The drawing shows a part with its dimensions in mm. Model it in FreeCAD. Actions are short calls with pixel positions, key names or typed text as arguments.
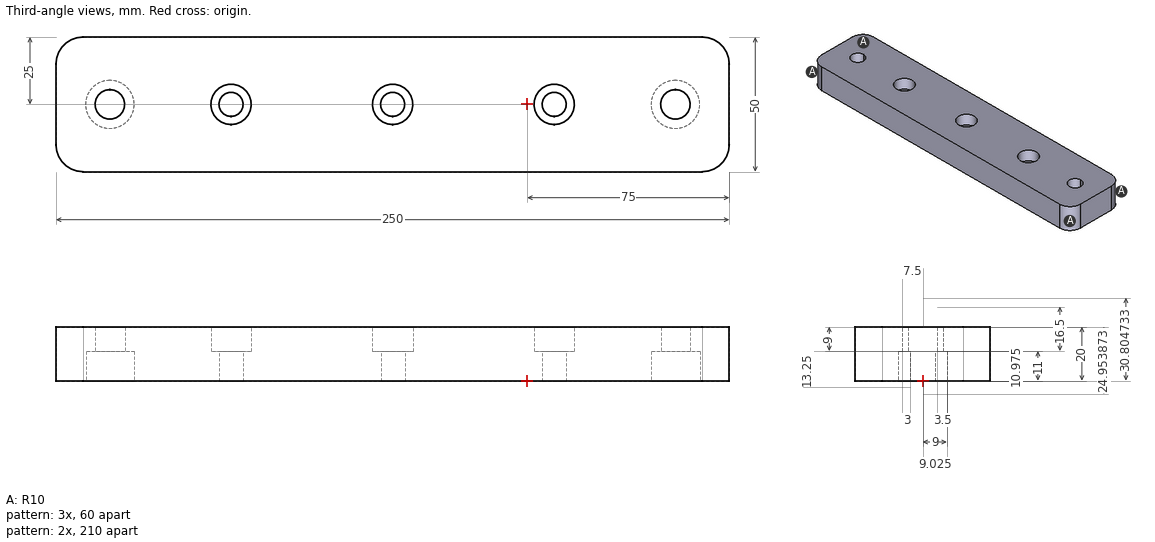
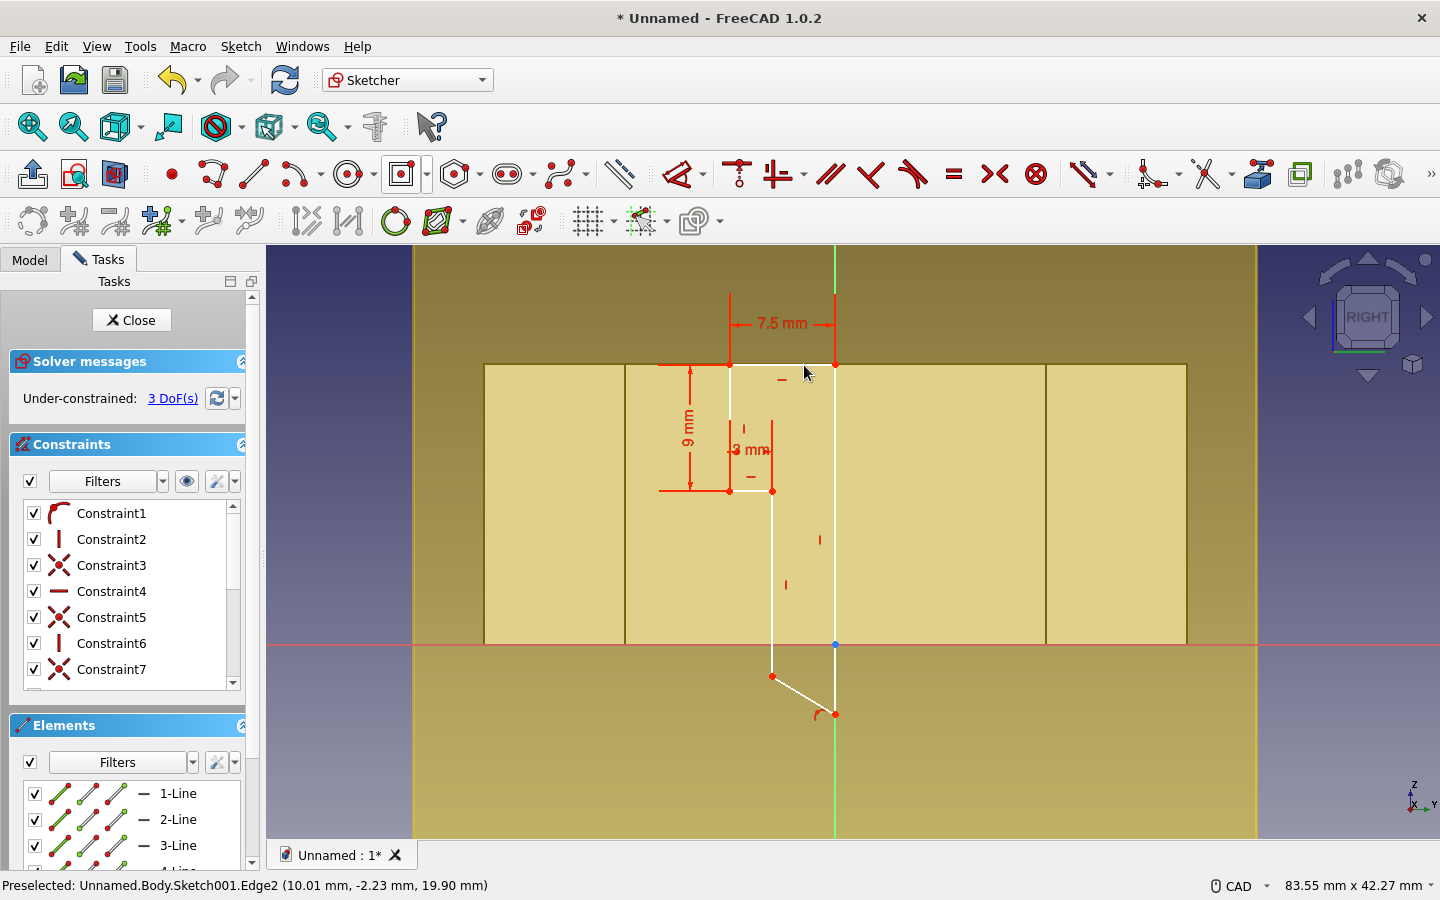
click(835, 365)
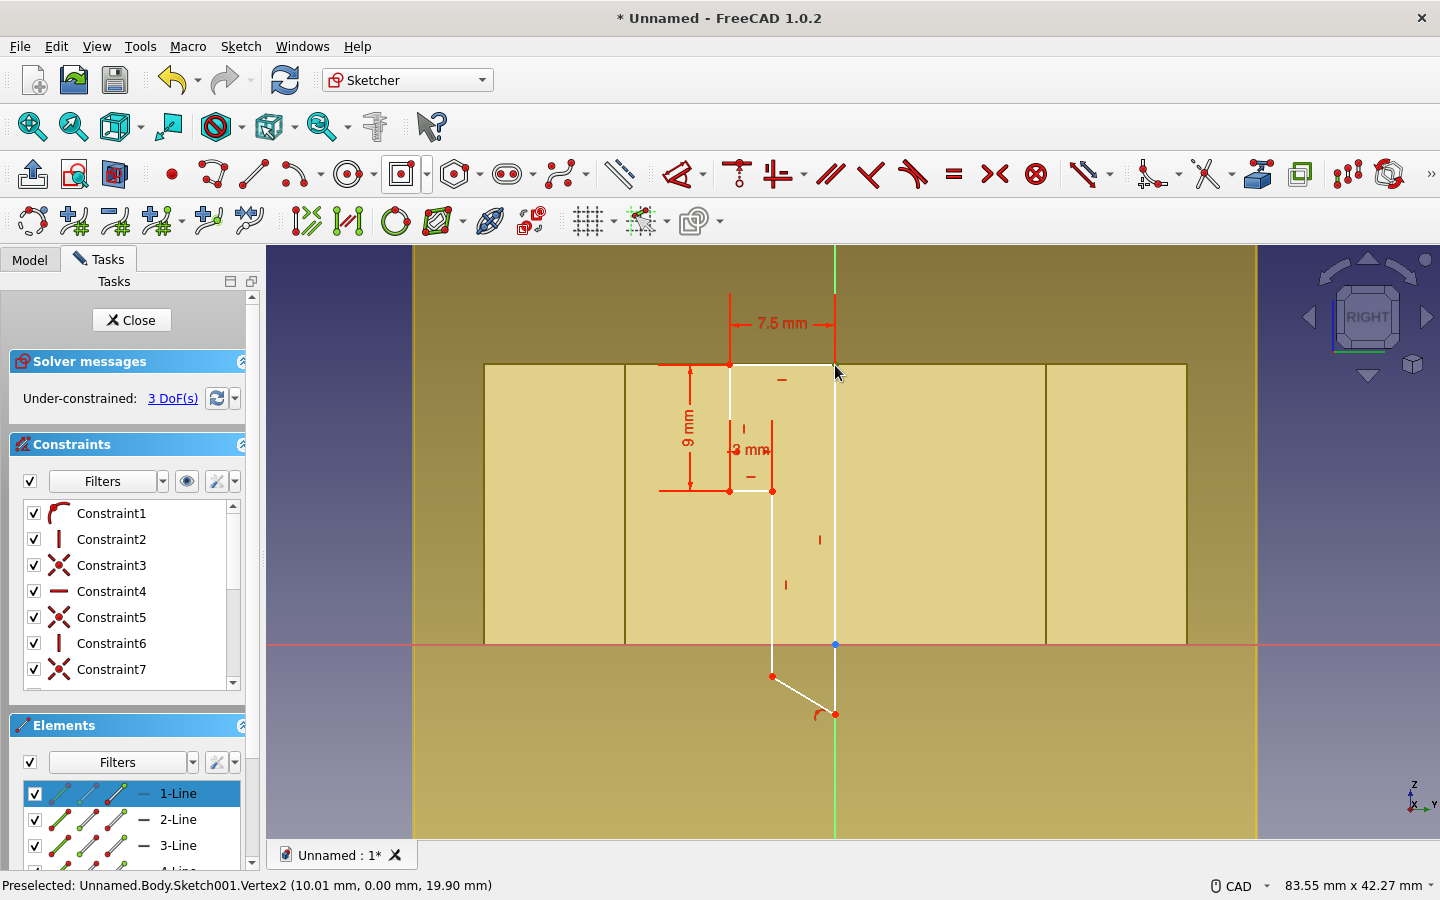
click(702, 174)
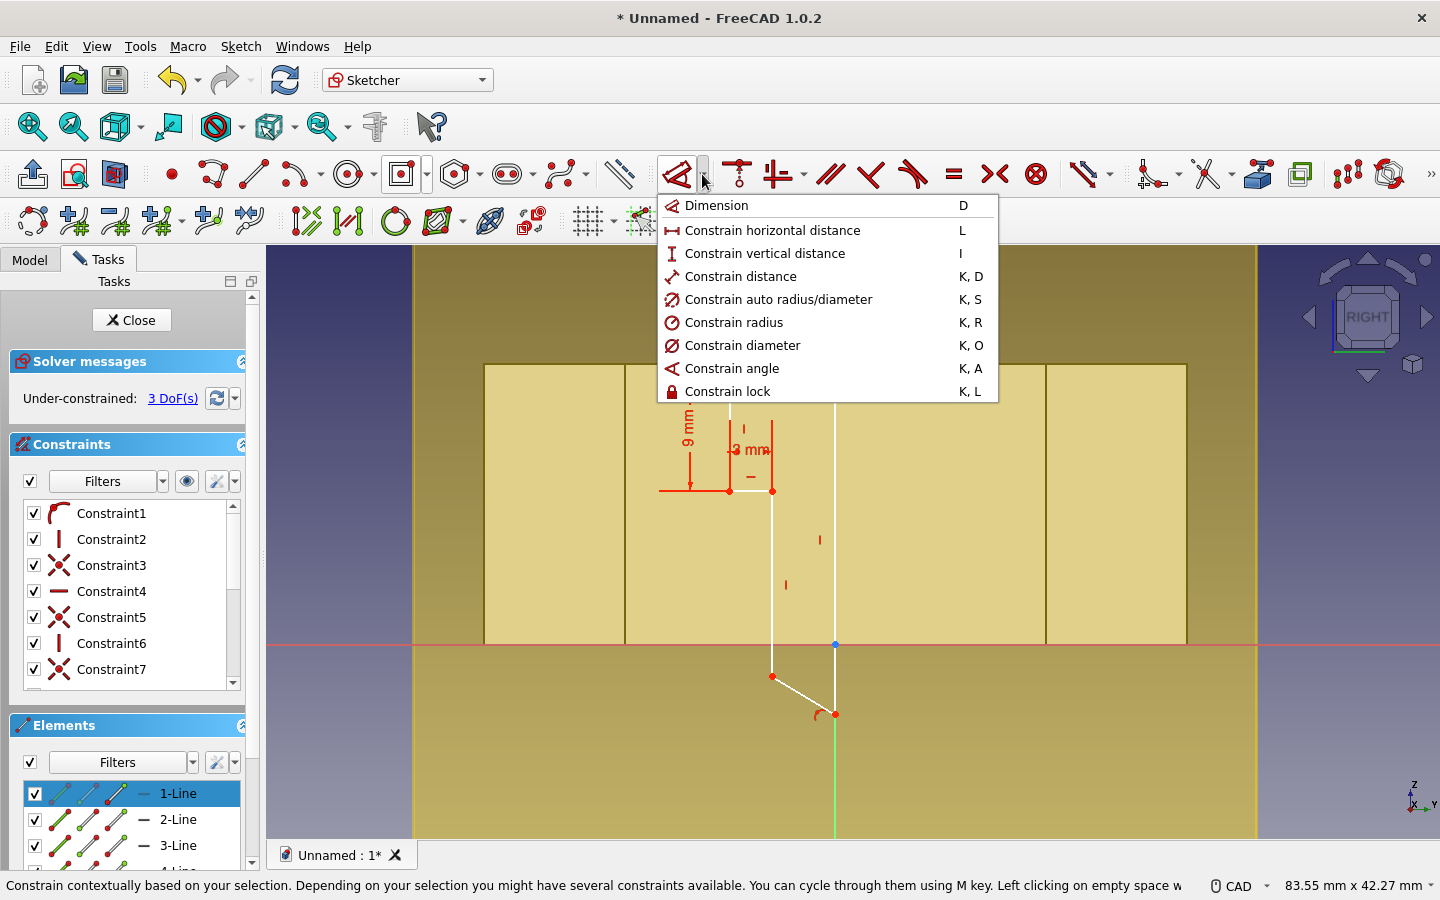
click(828, 254)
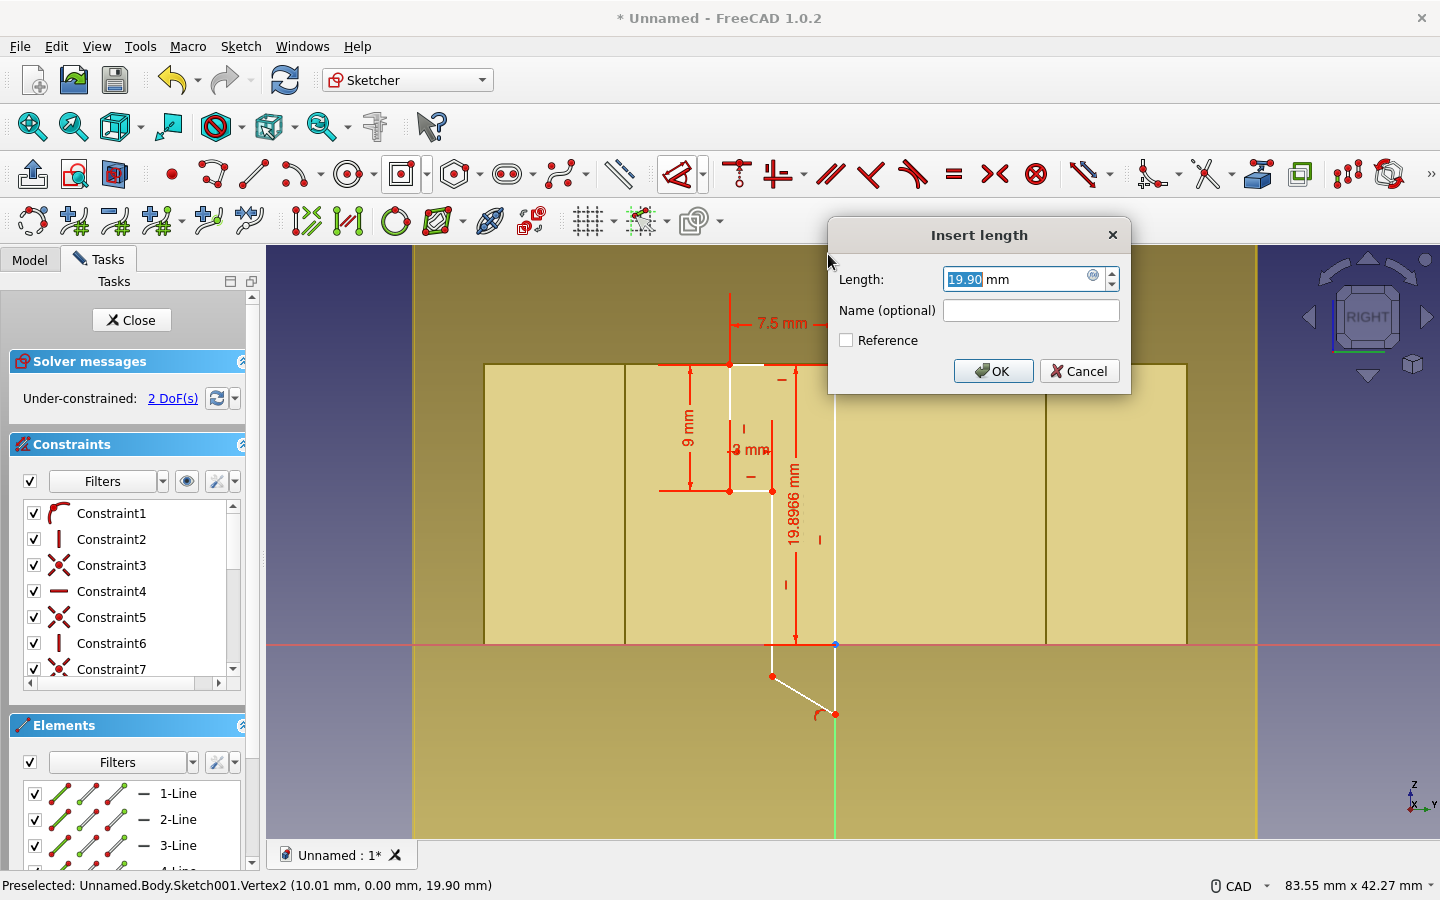
text(20)
key(Return)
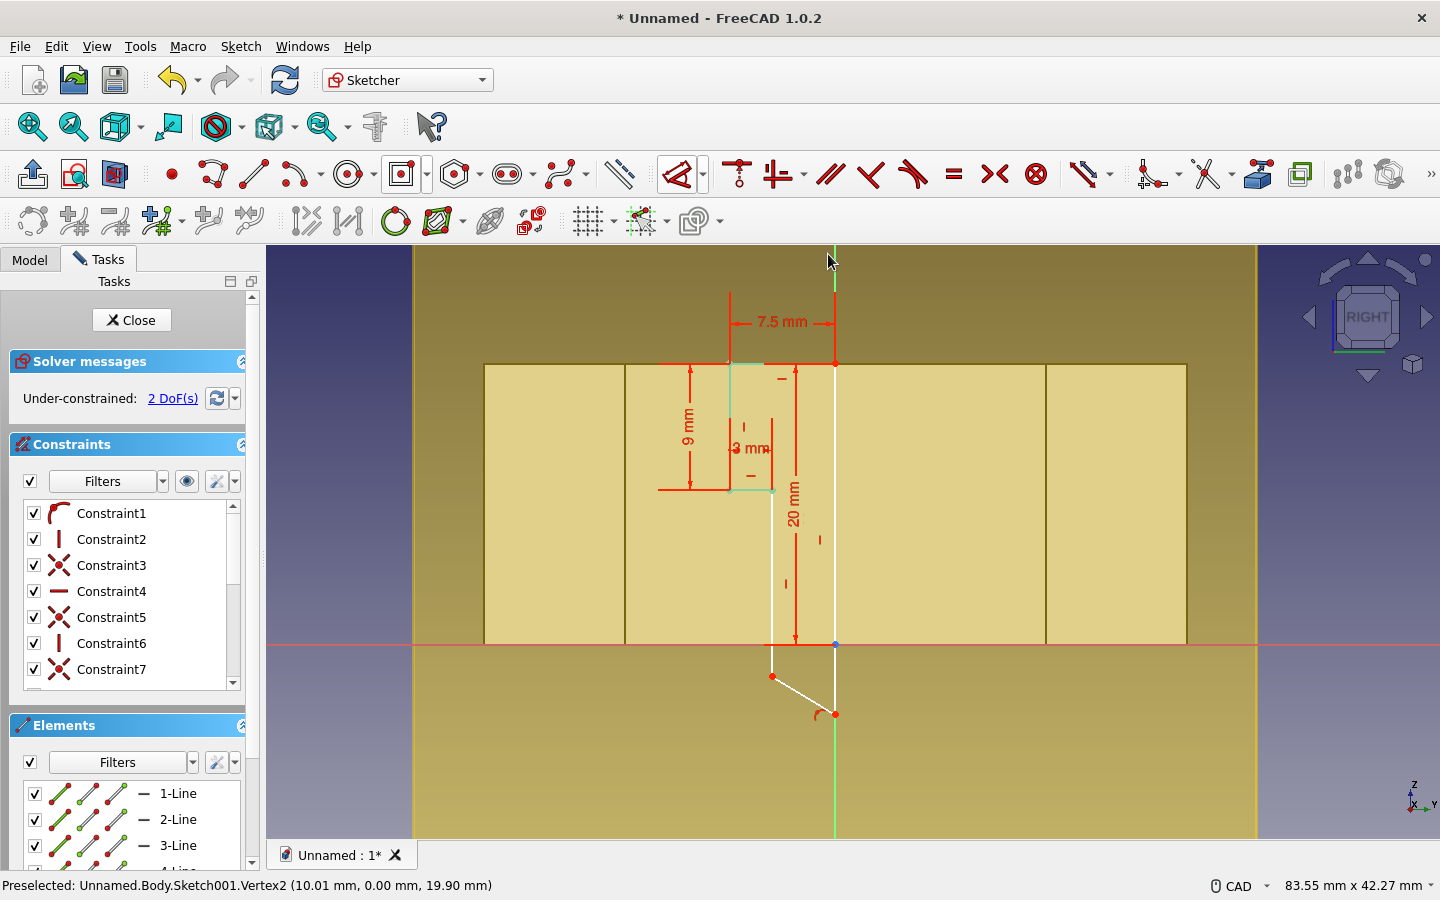
click(772, 546)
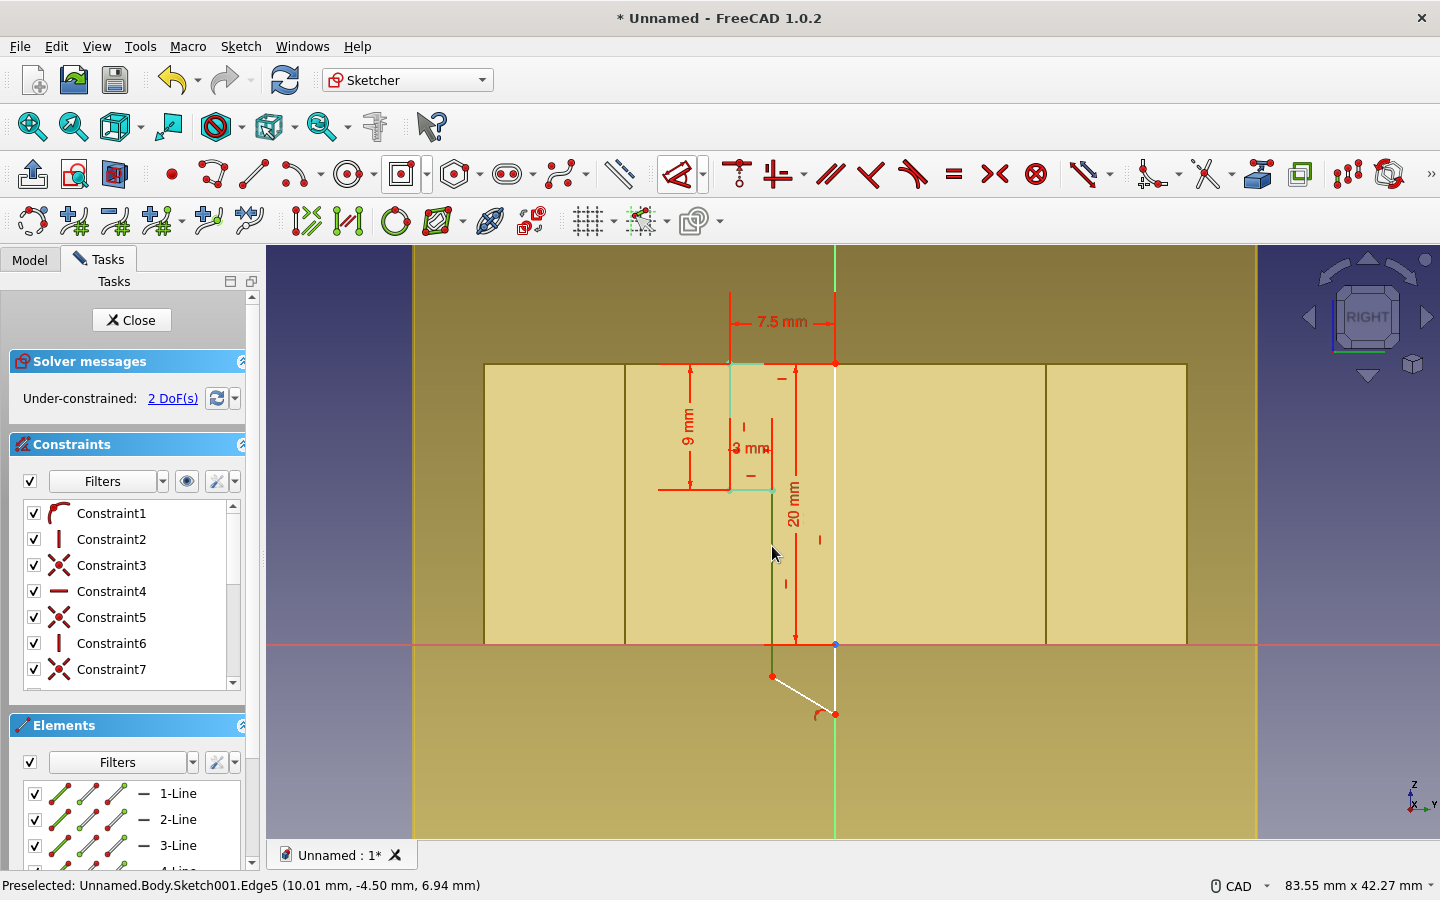
key(i)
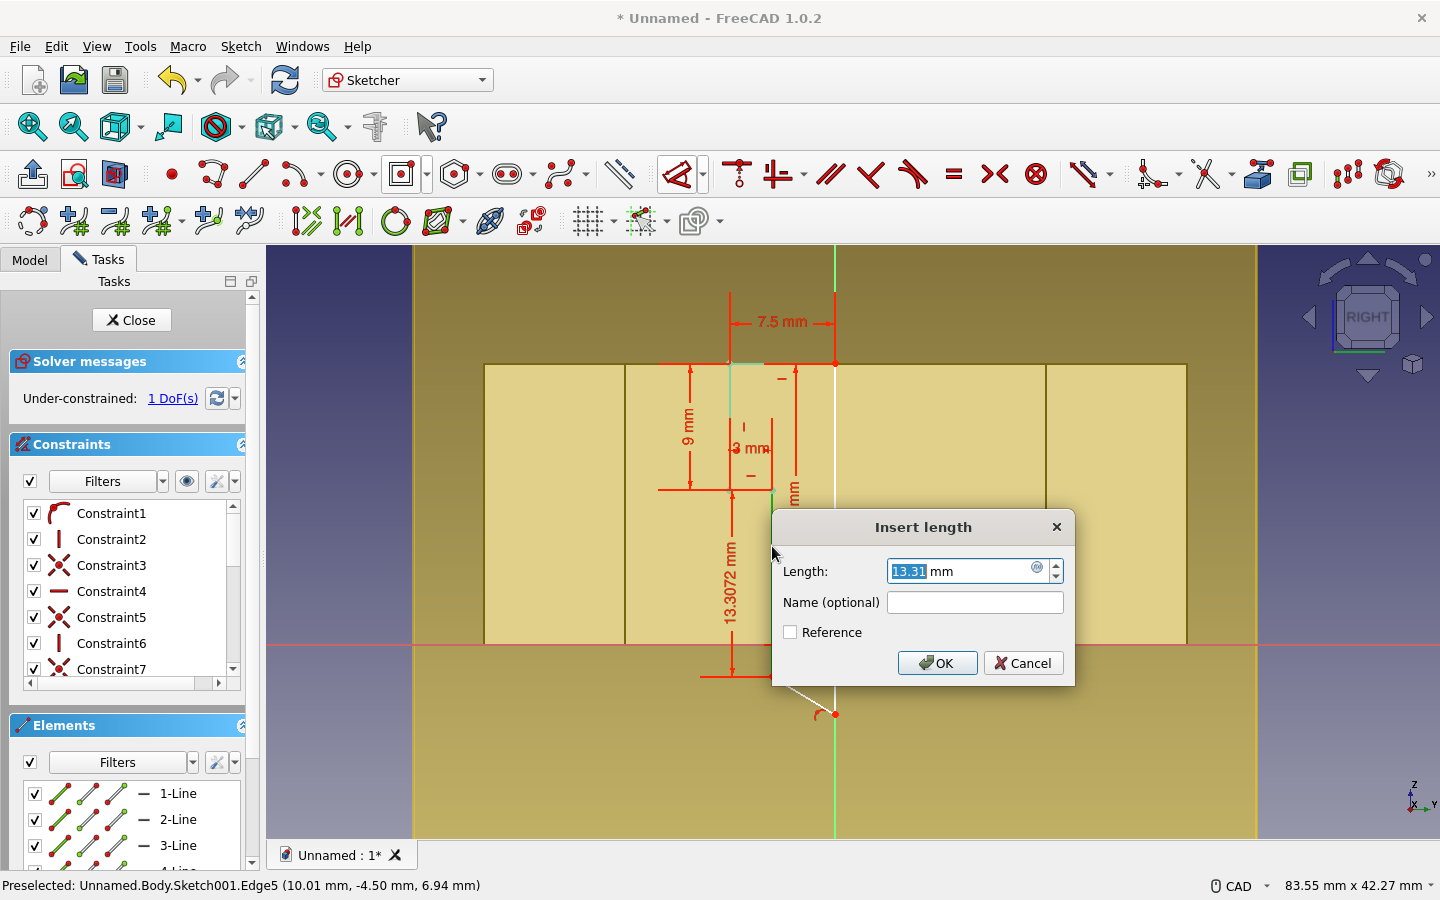
text(13.25)
key(Return)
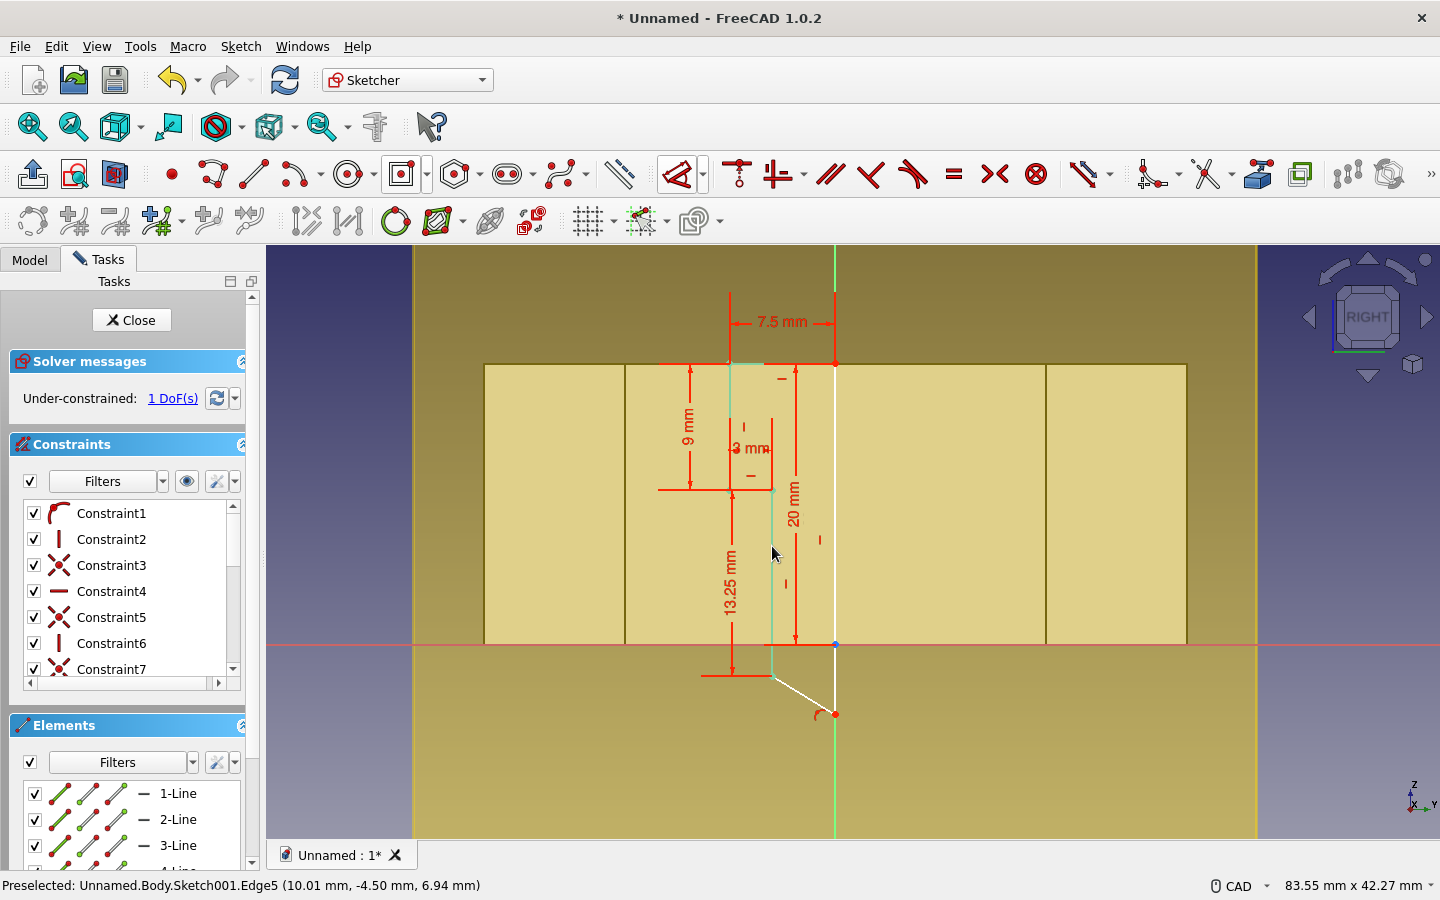
click(835, 610)